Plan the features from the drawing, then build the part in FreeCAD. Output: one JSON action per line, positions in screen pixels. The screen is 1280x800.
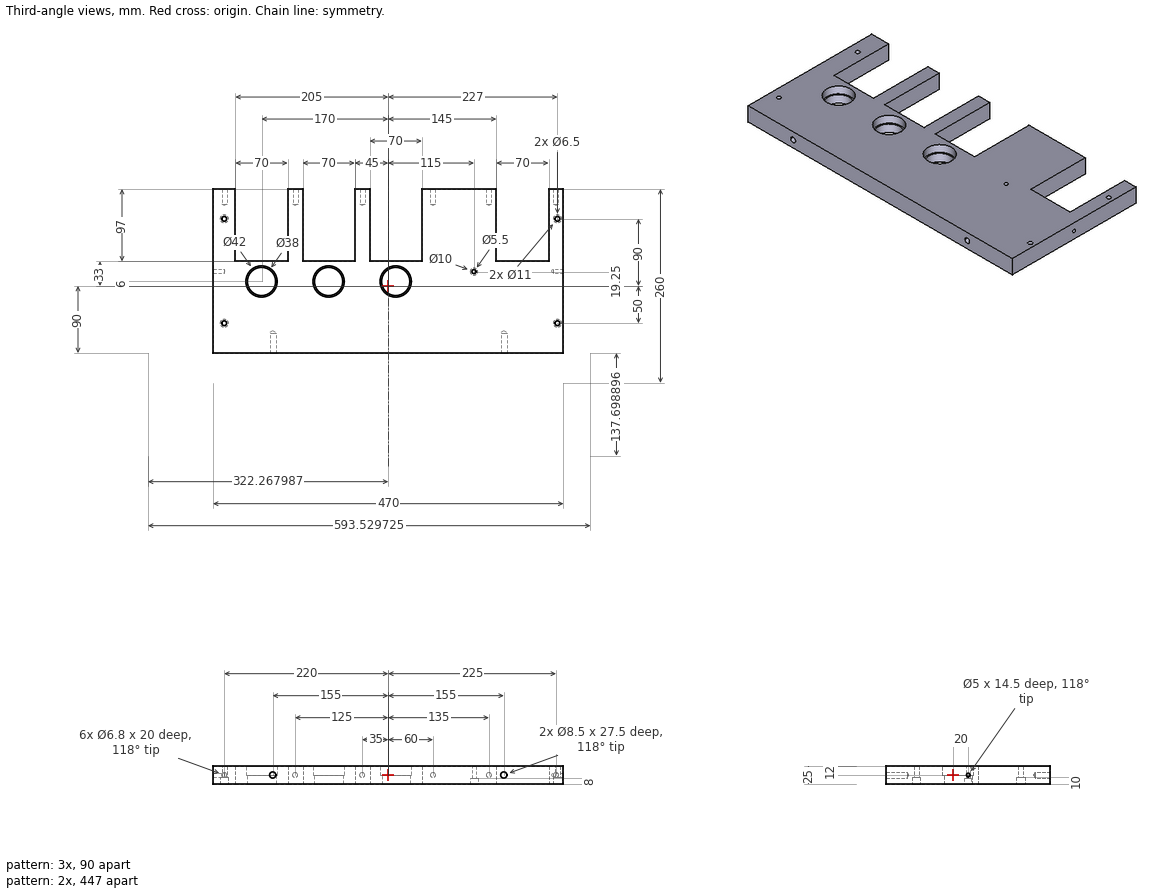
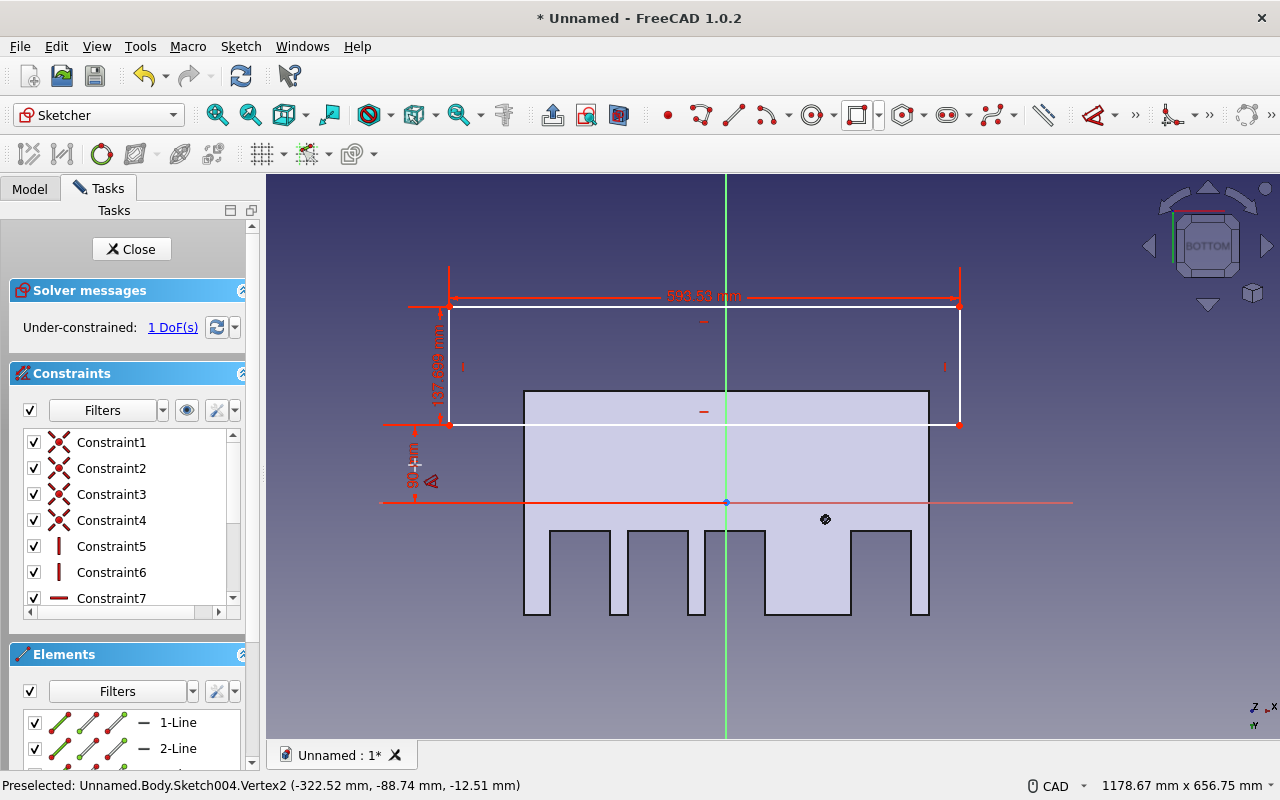
{"action": "left_click", "coordinate": [449, 307]}
{"action": "left_click", "coordinate": [588, 537]}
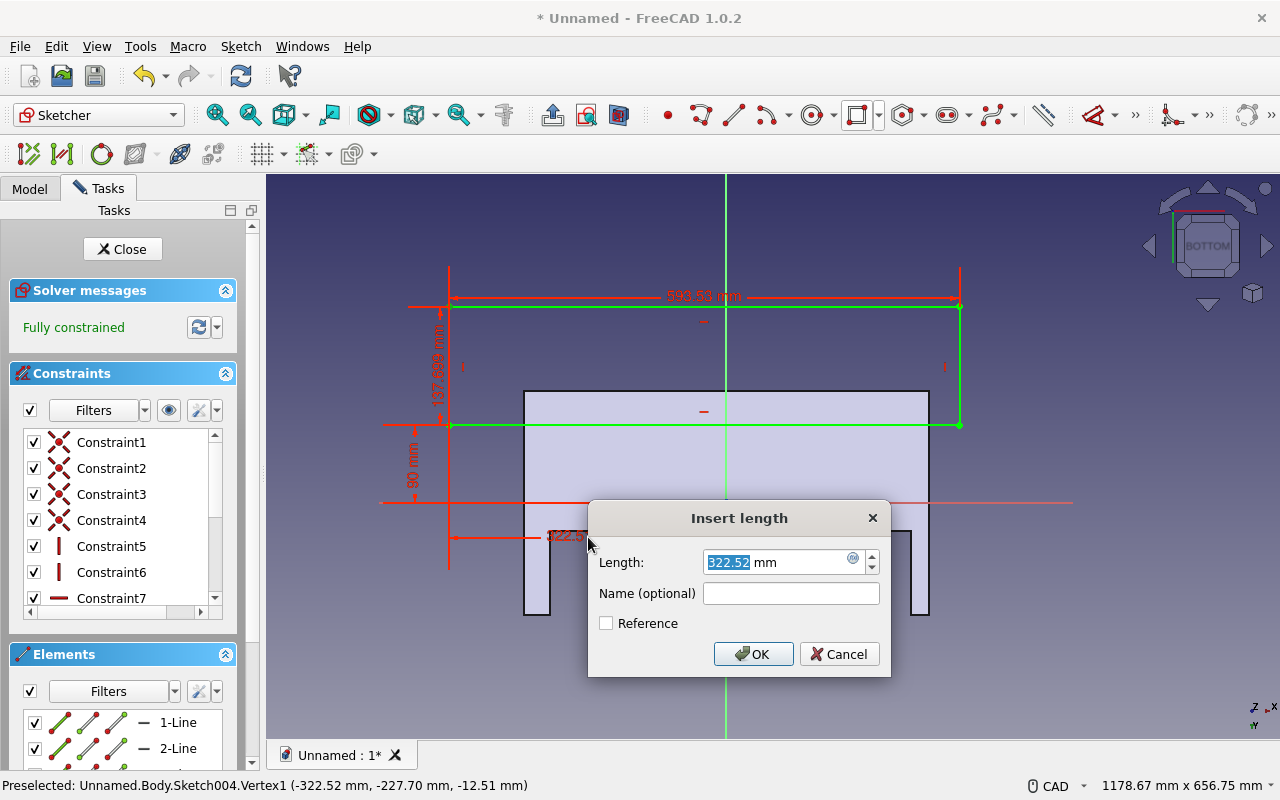
{"action": "type", "text": "322.267987"}
{"action": "key", "text": "Return"}
{"action": "key", "text": "Escape"}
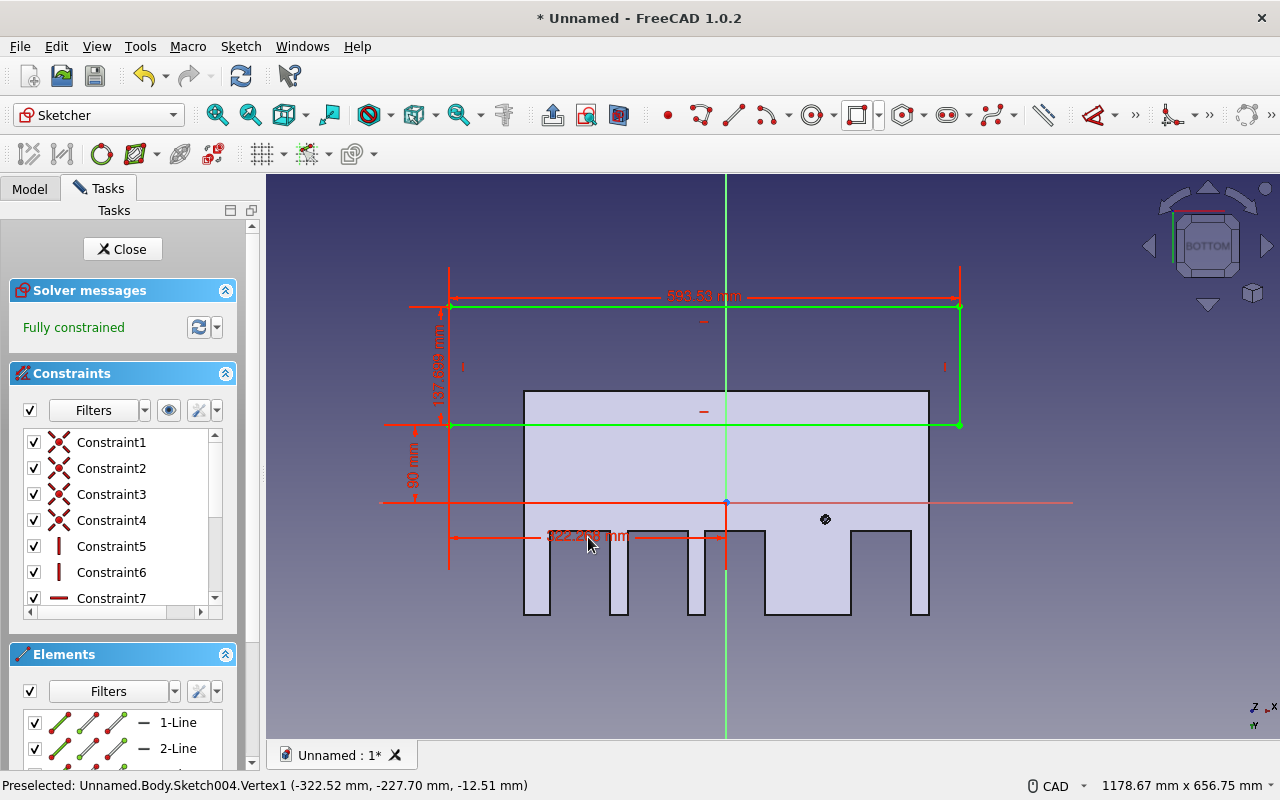
{"action": "left_click", "coordinate": [123, 249]}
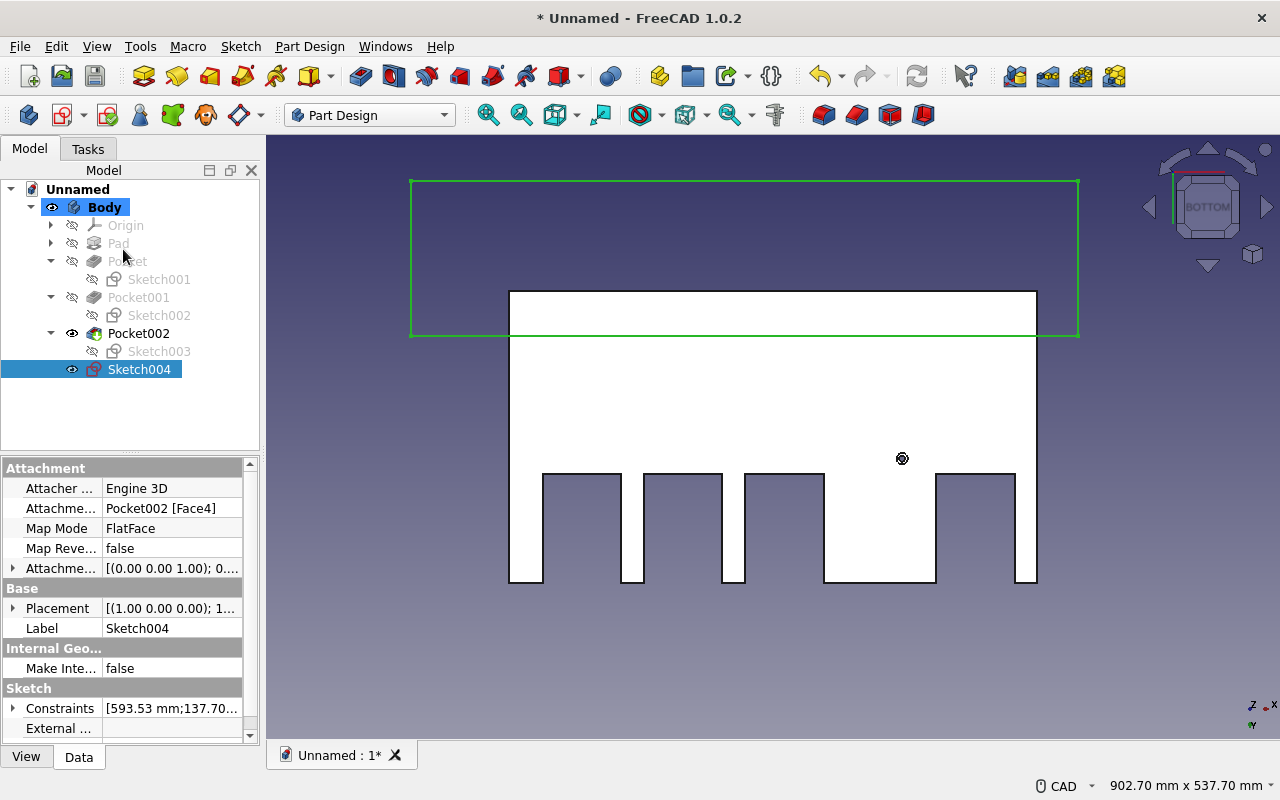
{"action": "left_click", "coordinate": [361, 76]}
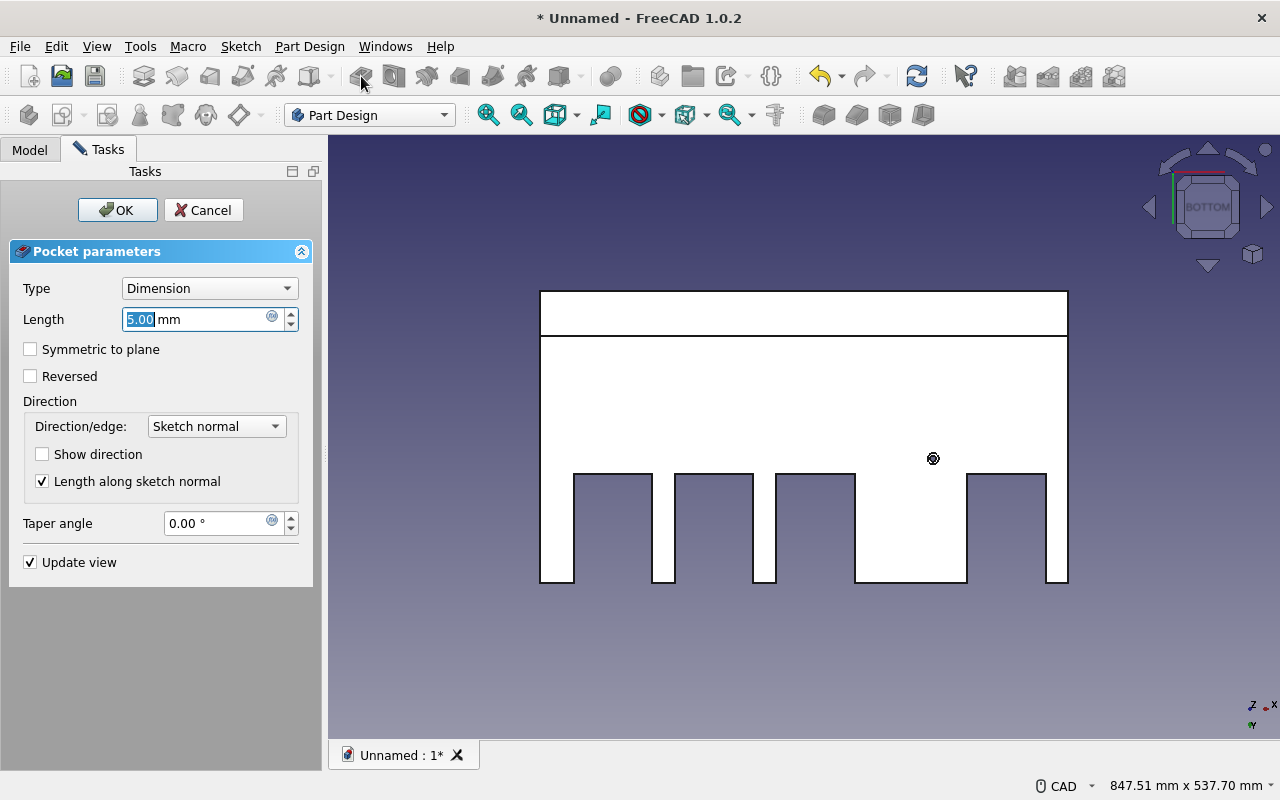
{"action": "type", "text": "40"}
{"action": "key", "text": "Tab"}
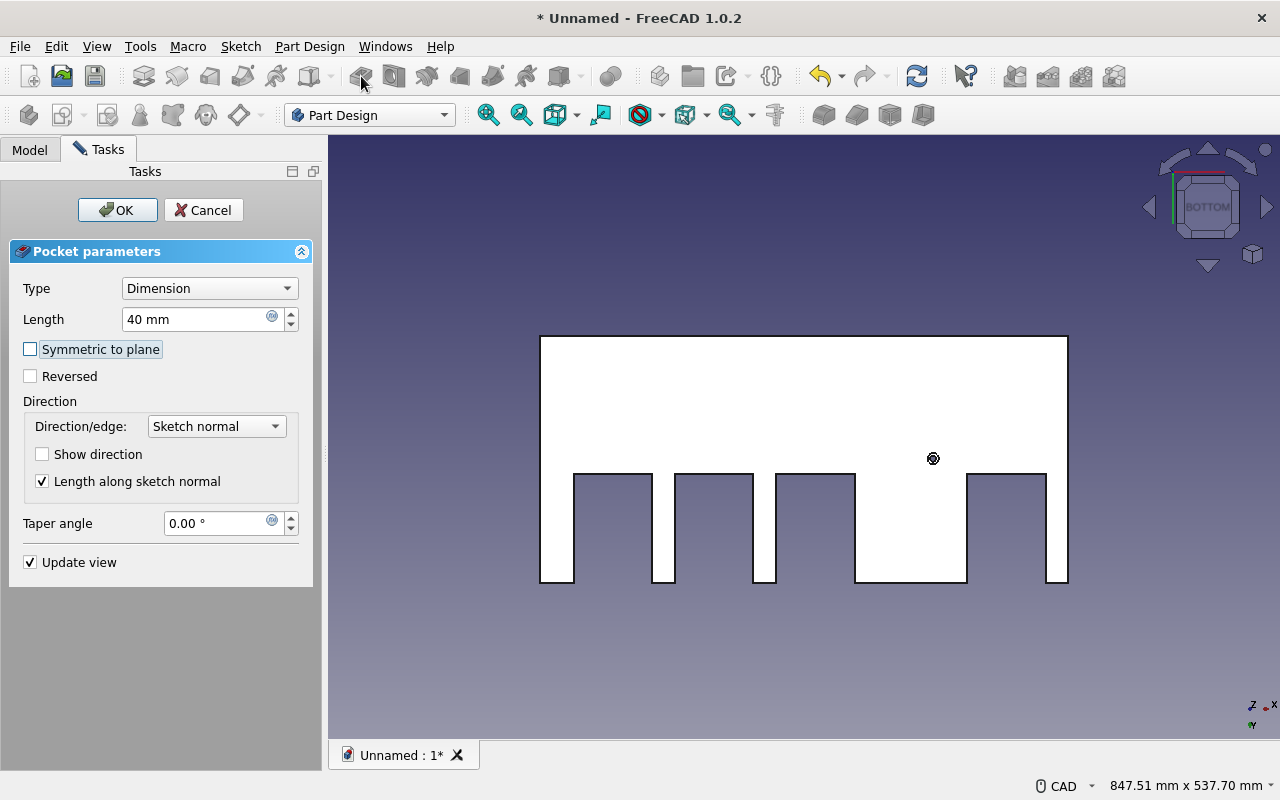
{"action": "left_click", "coordinate": [118, 210]}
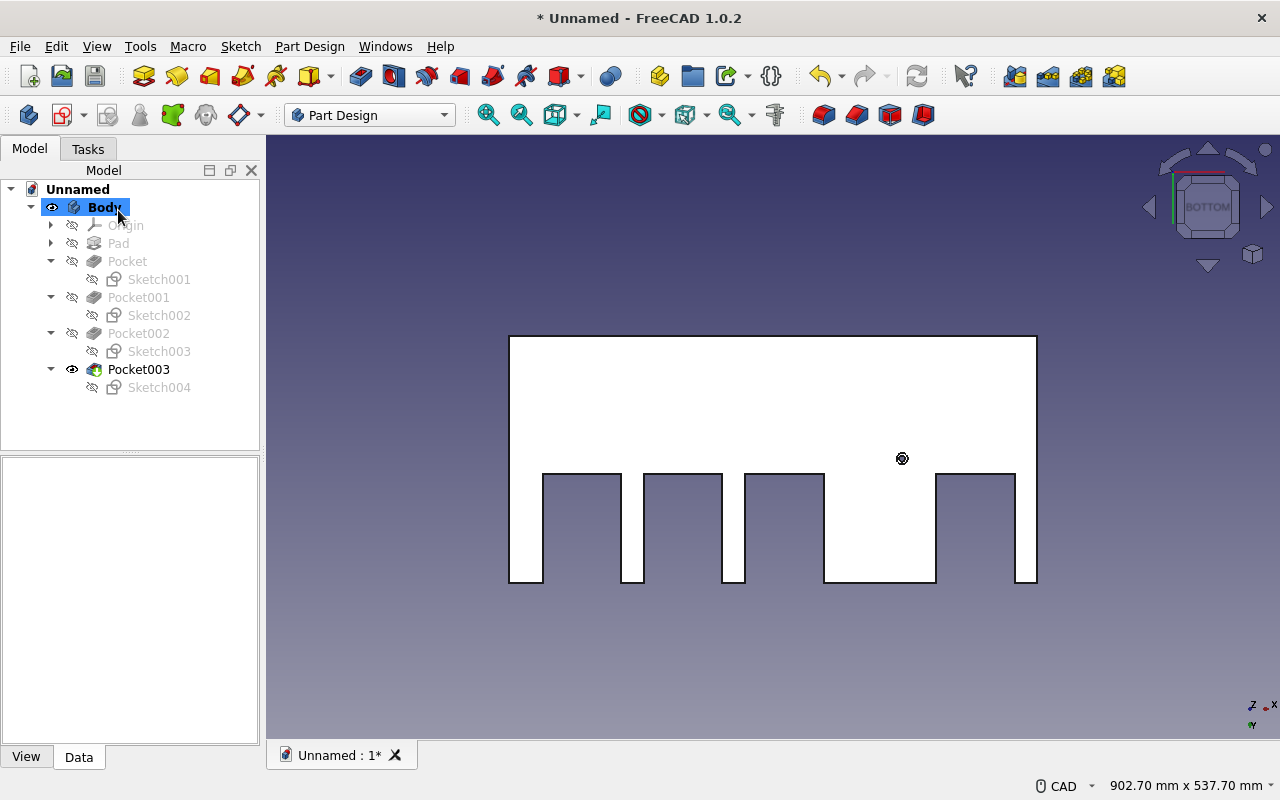
{"action": "key", "text": "4"}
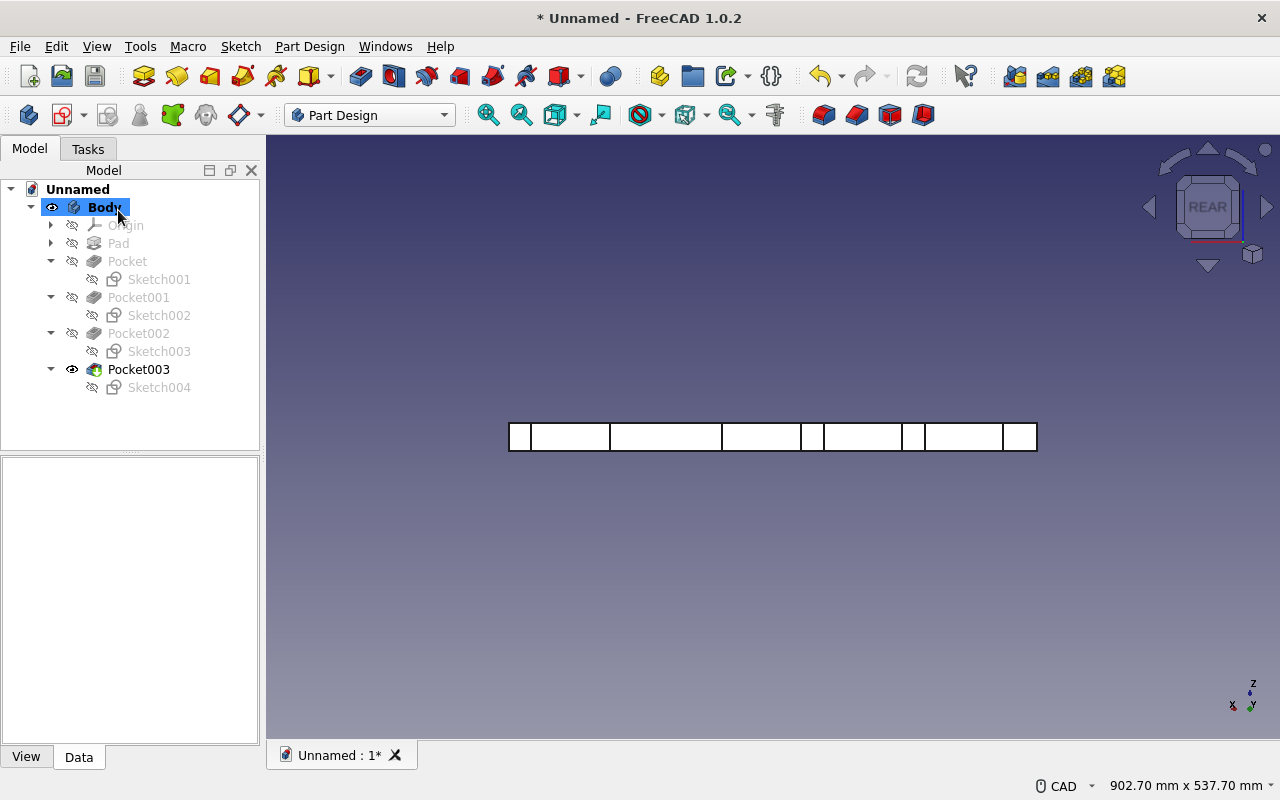
{"action": "left_click", "coordinate": [634, 436]}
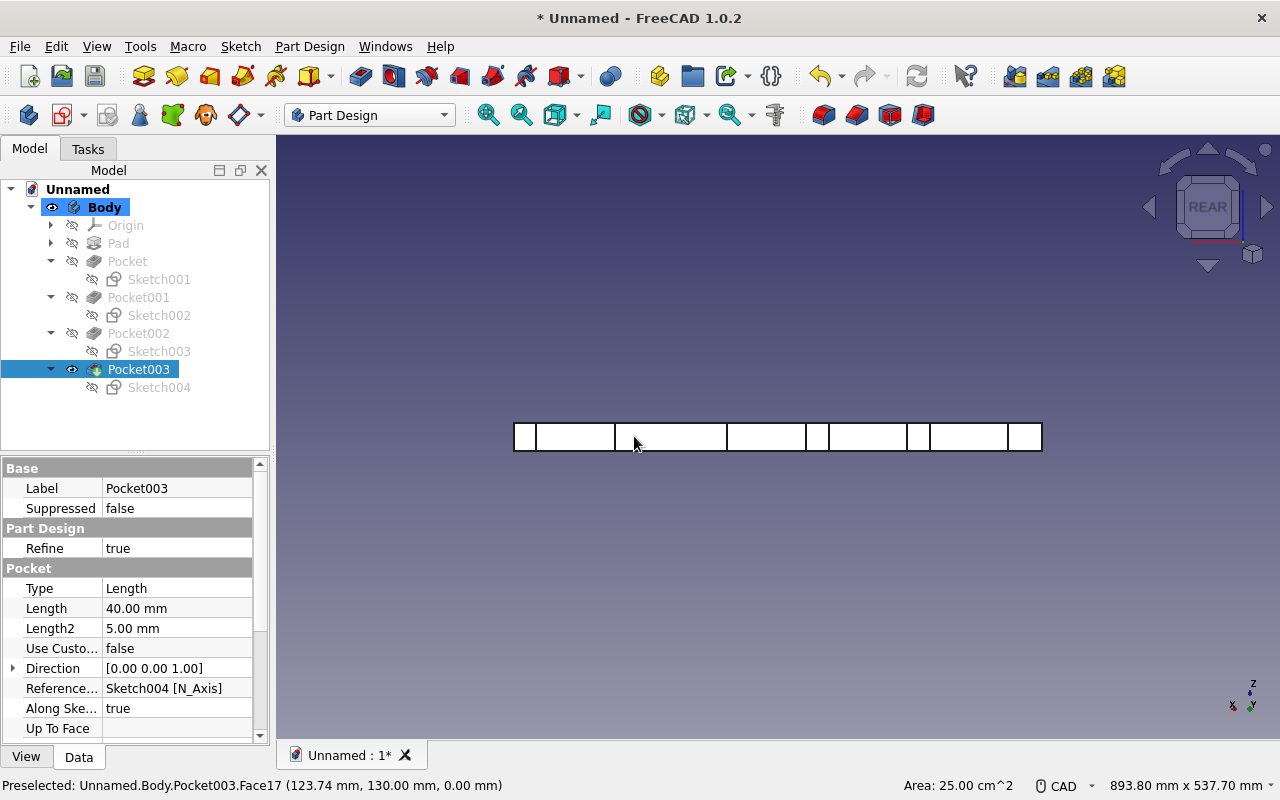
{"action": "left_click", "coordinate": [62, 116]}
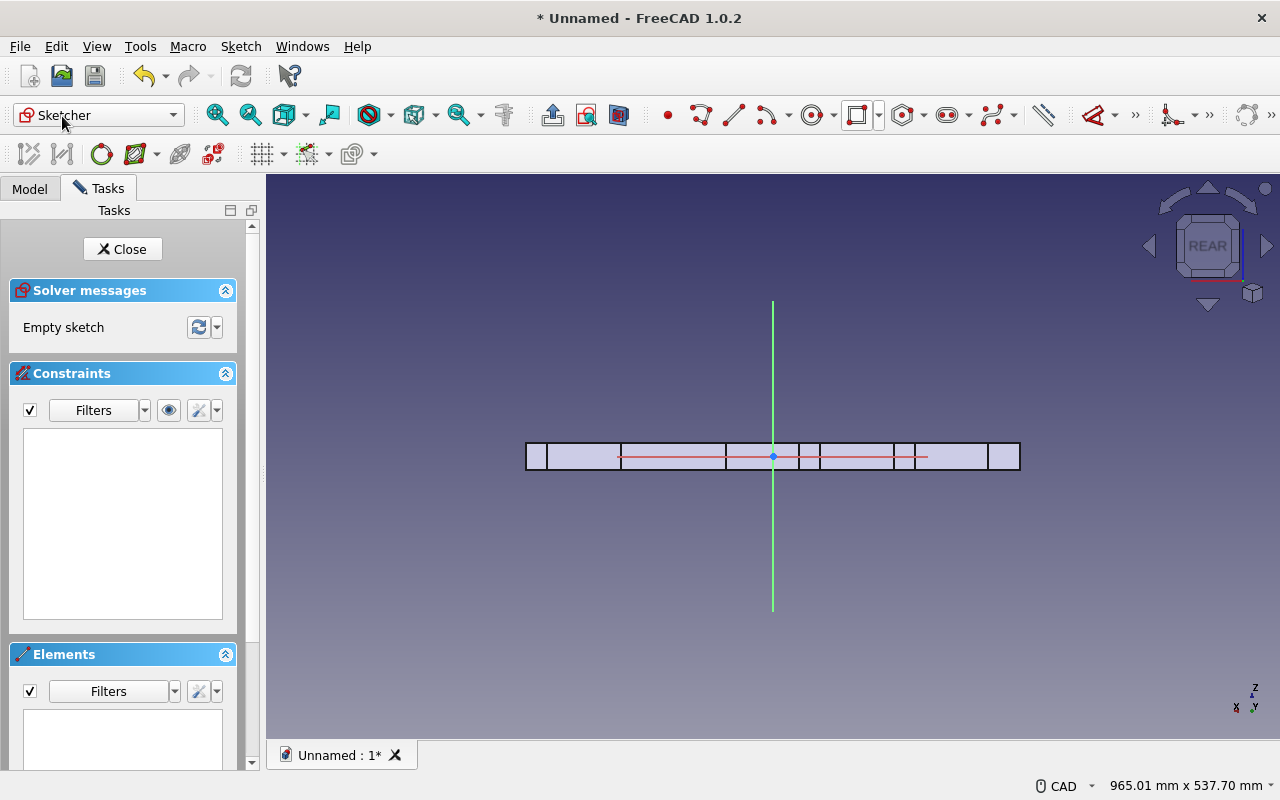
{"action": "left_click", "coordinate": [812, 116]}